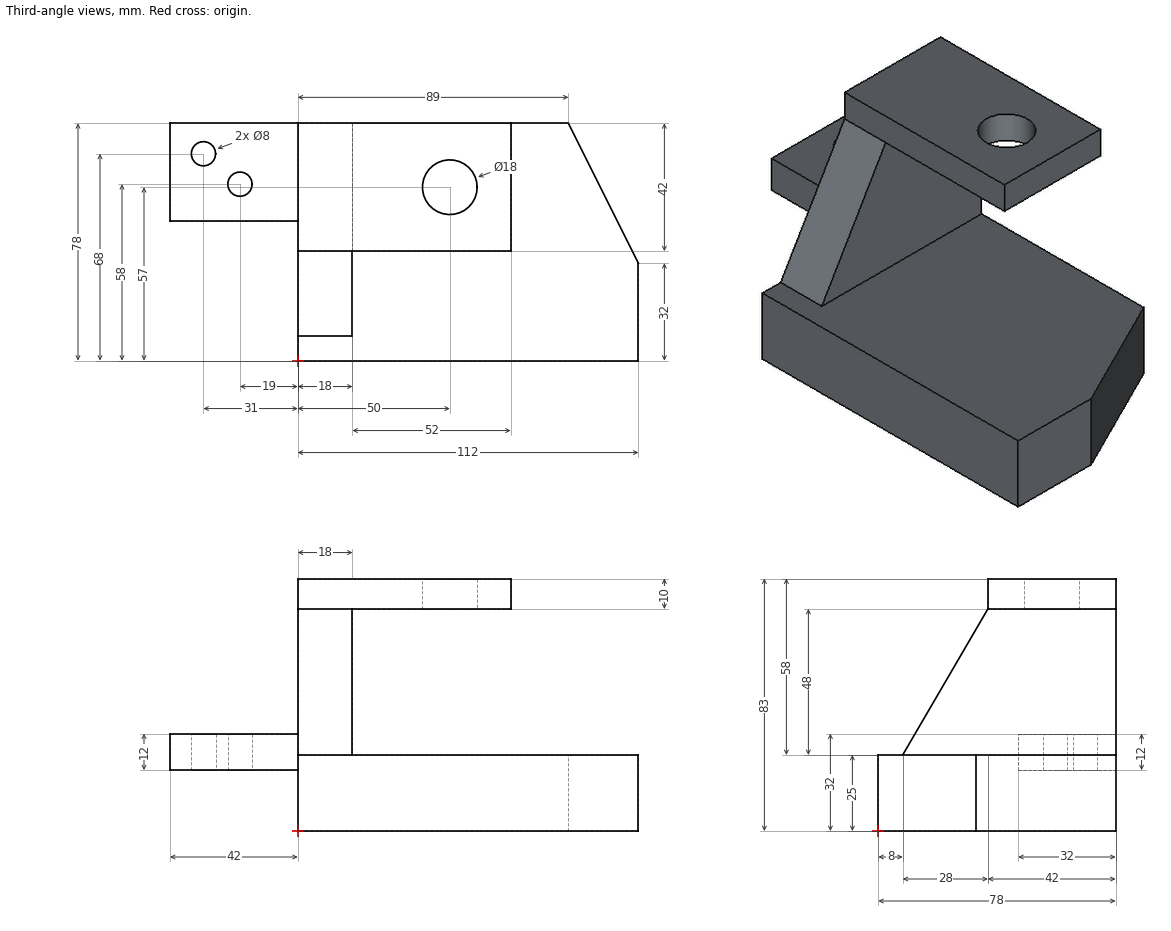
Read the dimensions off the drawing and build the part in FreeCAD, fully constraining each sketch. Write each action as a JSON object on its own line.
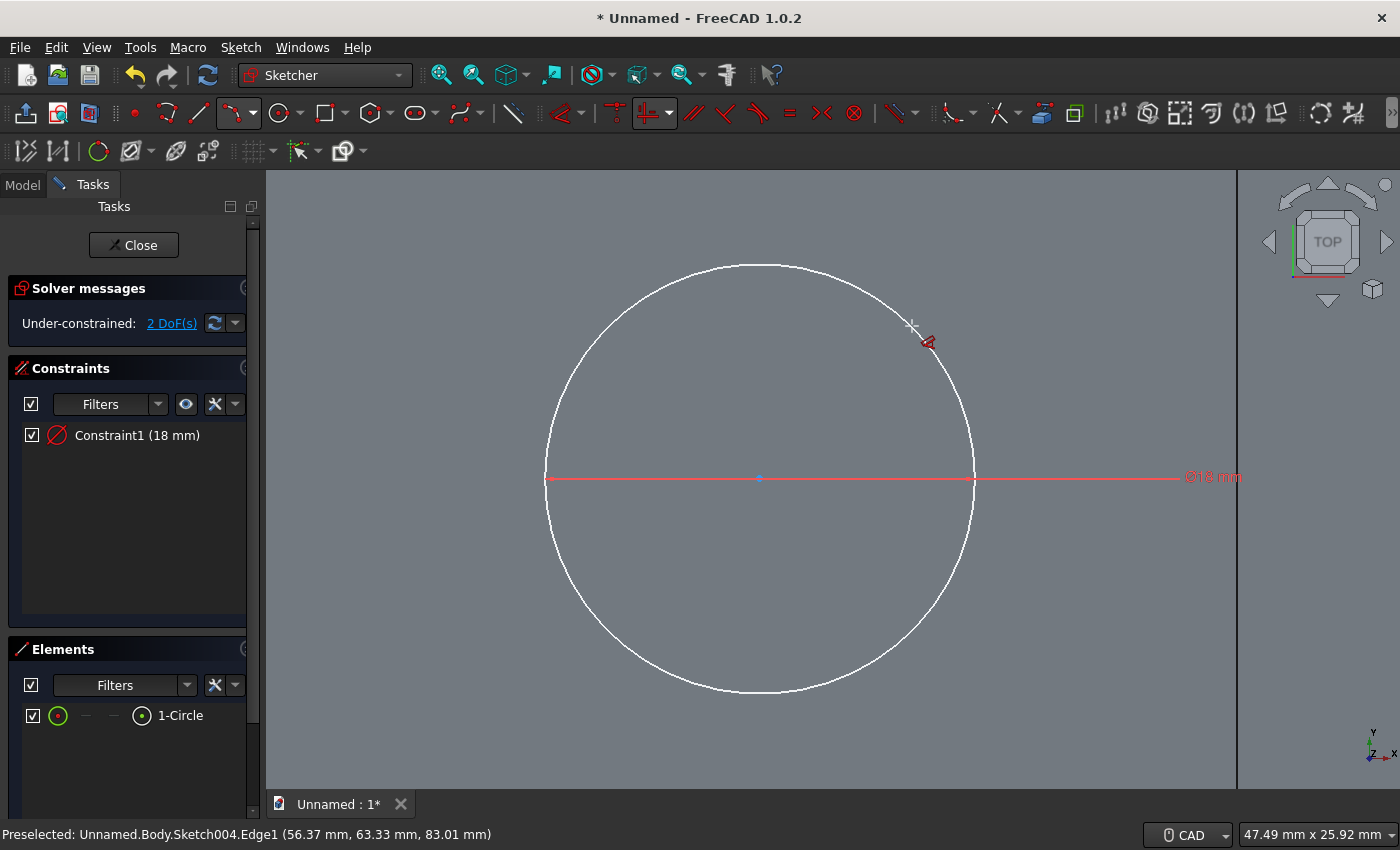
{"action": "left_click", "coordinate": [760, 479]}
{"action": "left_click", "coordinate": [527, 445]}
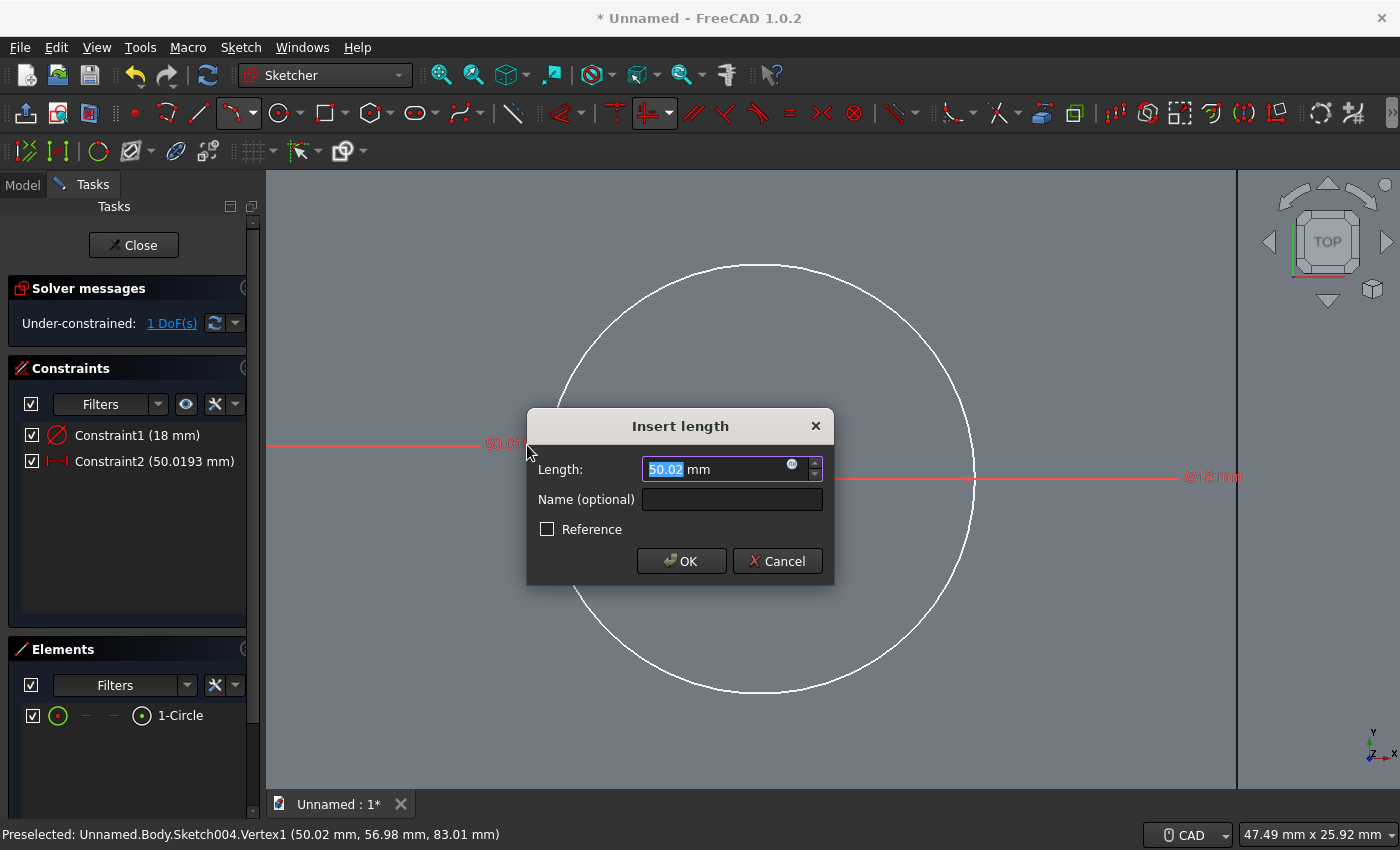
{"action": "type", "text": "50"}
{"action": "key", "text": "Return"}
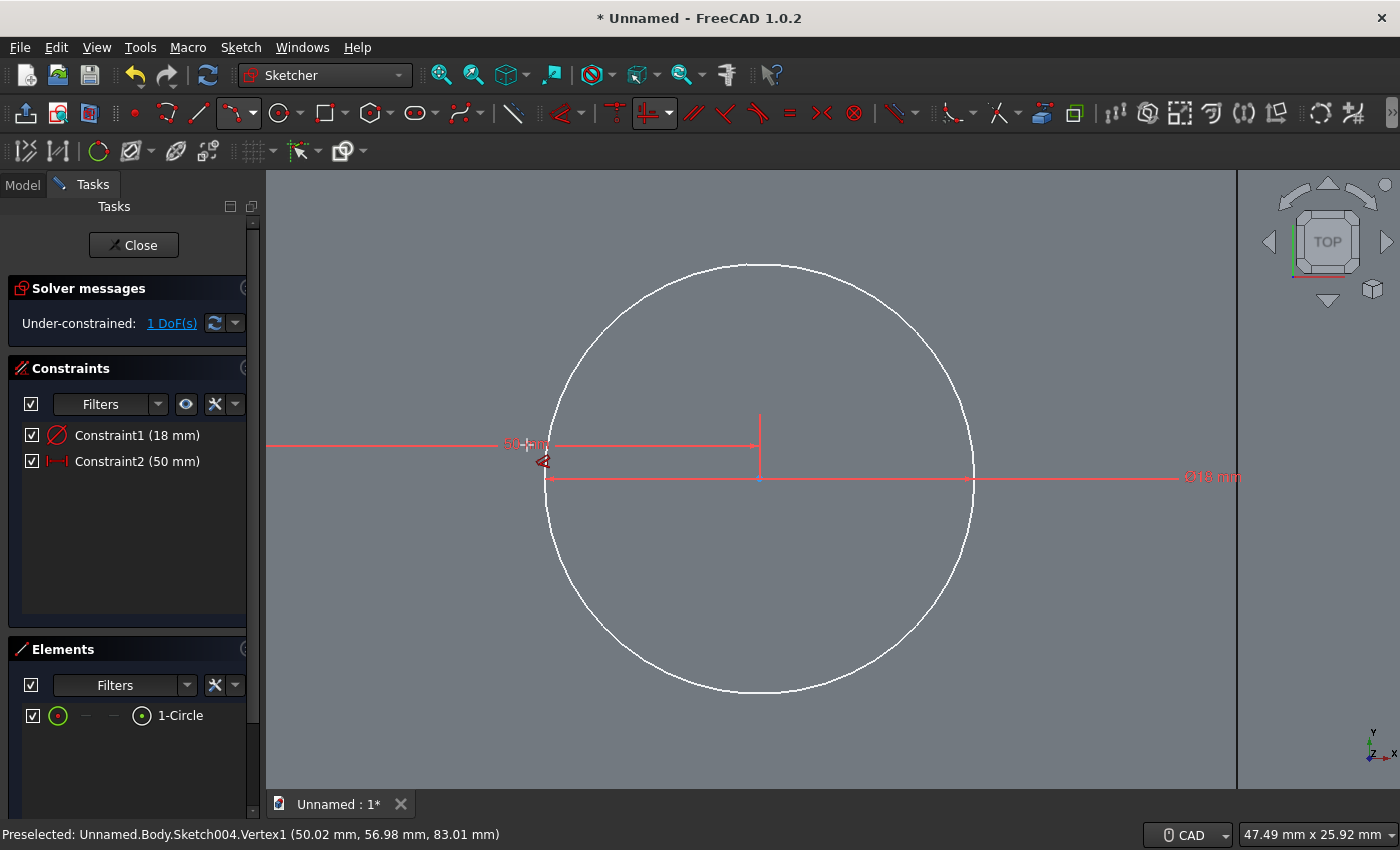
{"action": "left_click", "coordinate": [760, 479]}
{"action": "left_click", "coordinate": [794, 620]}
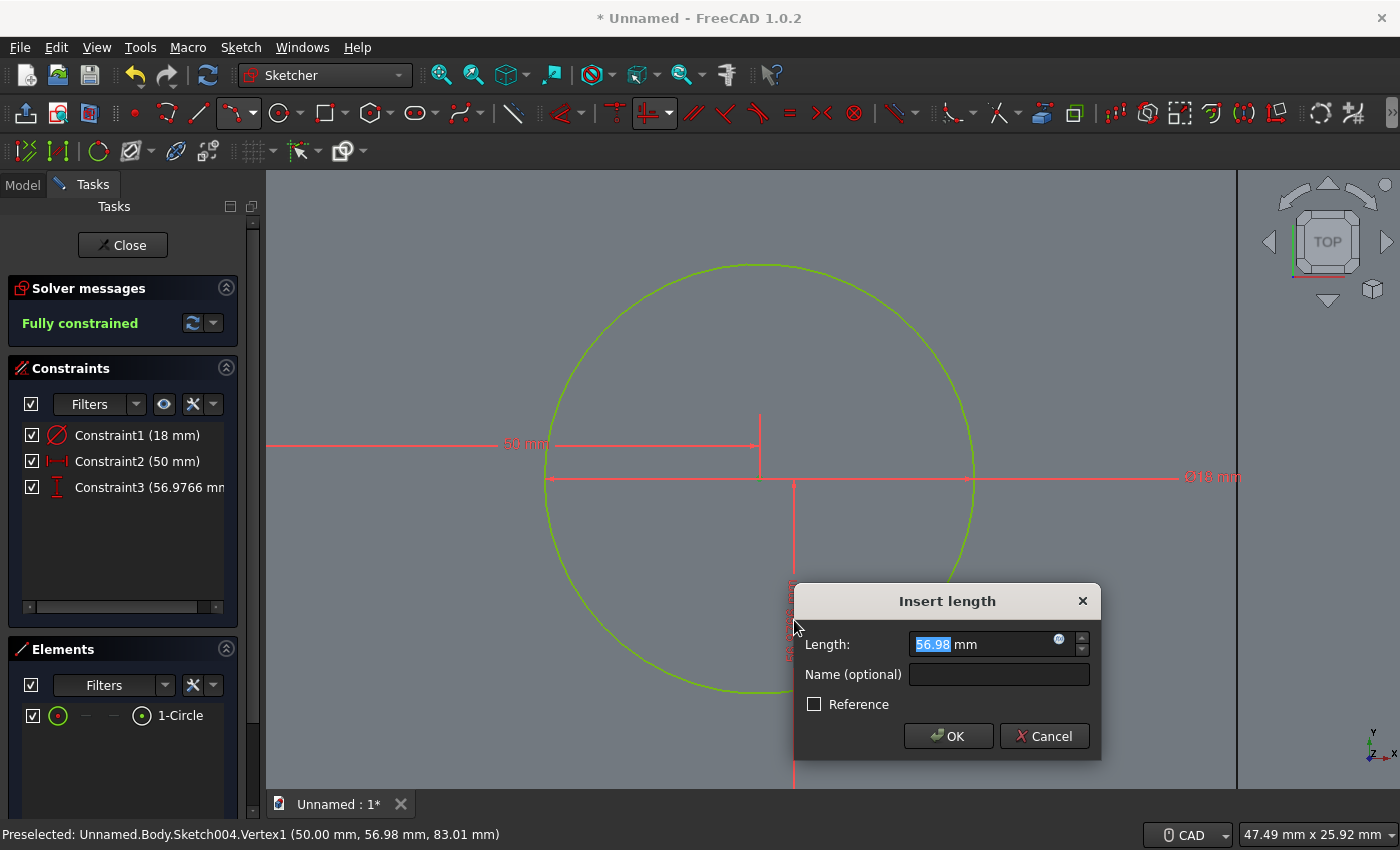
{"action": "type", "text": "57"}
{"action": "key", "text": "Return"}
{"action": "key", "text": "Escape"}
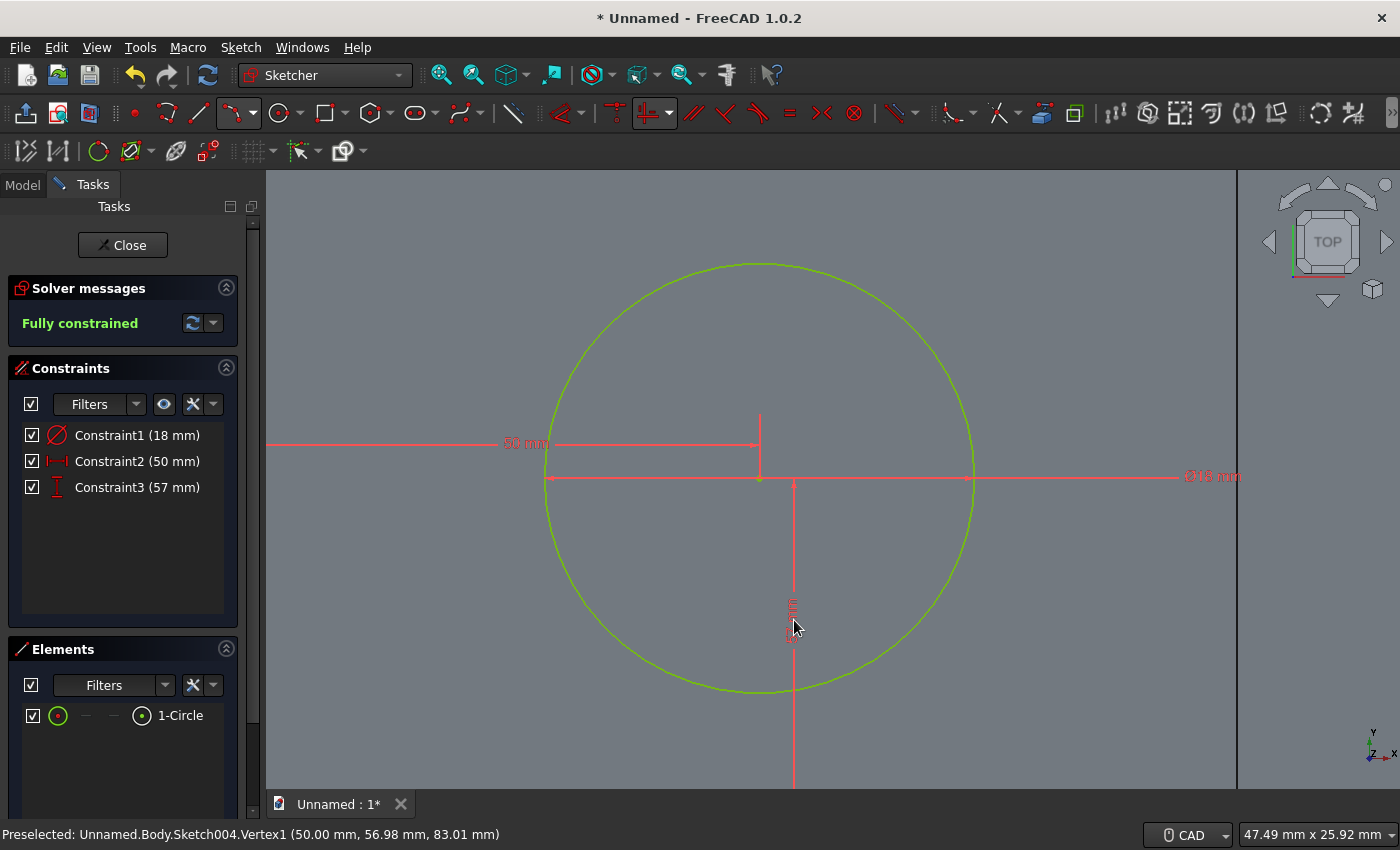
{"action": "left_click", "coordinate": [123, 245]}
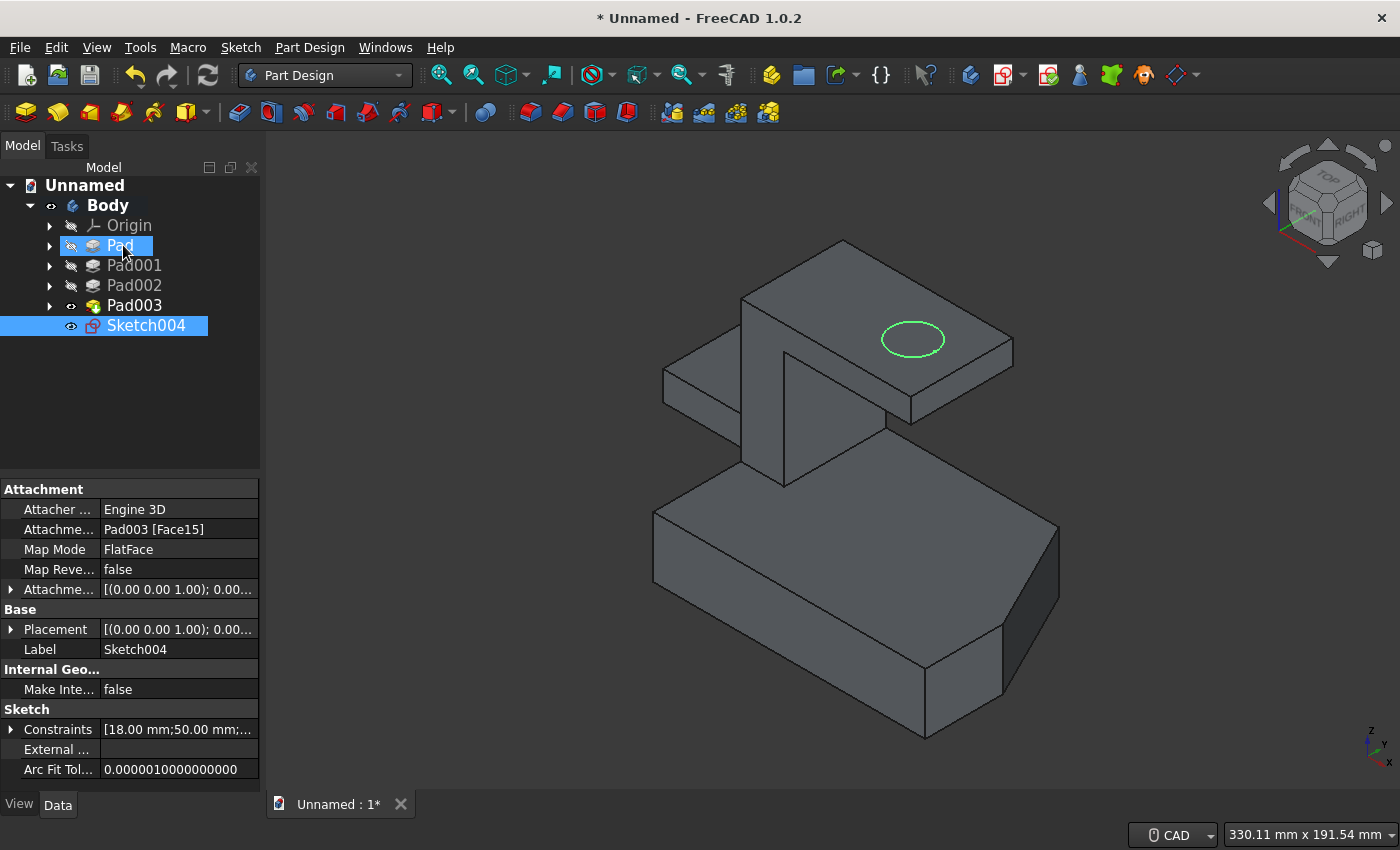
{"action": "left_click", "coordinate": [240, 112]}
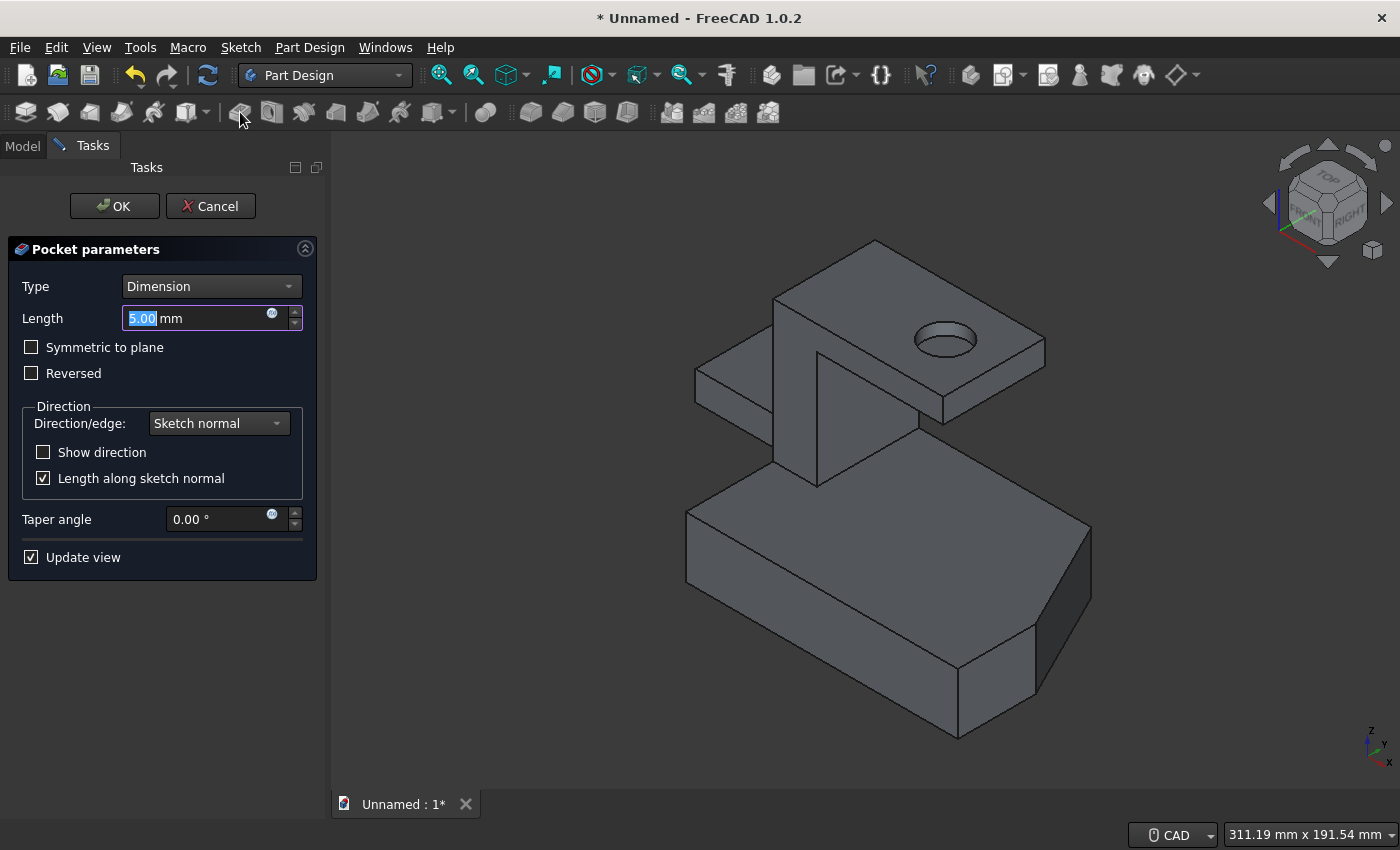
{"action": "type", "text": "10"}
{"action": "key", "text": "Tab"}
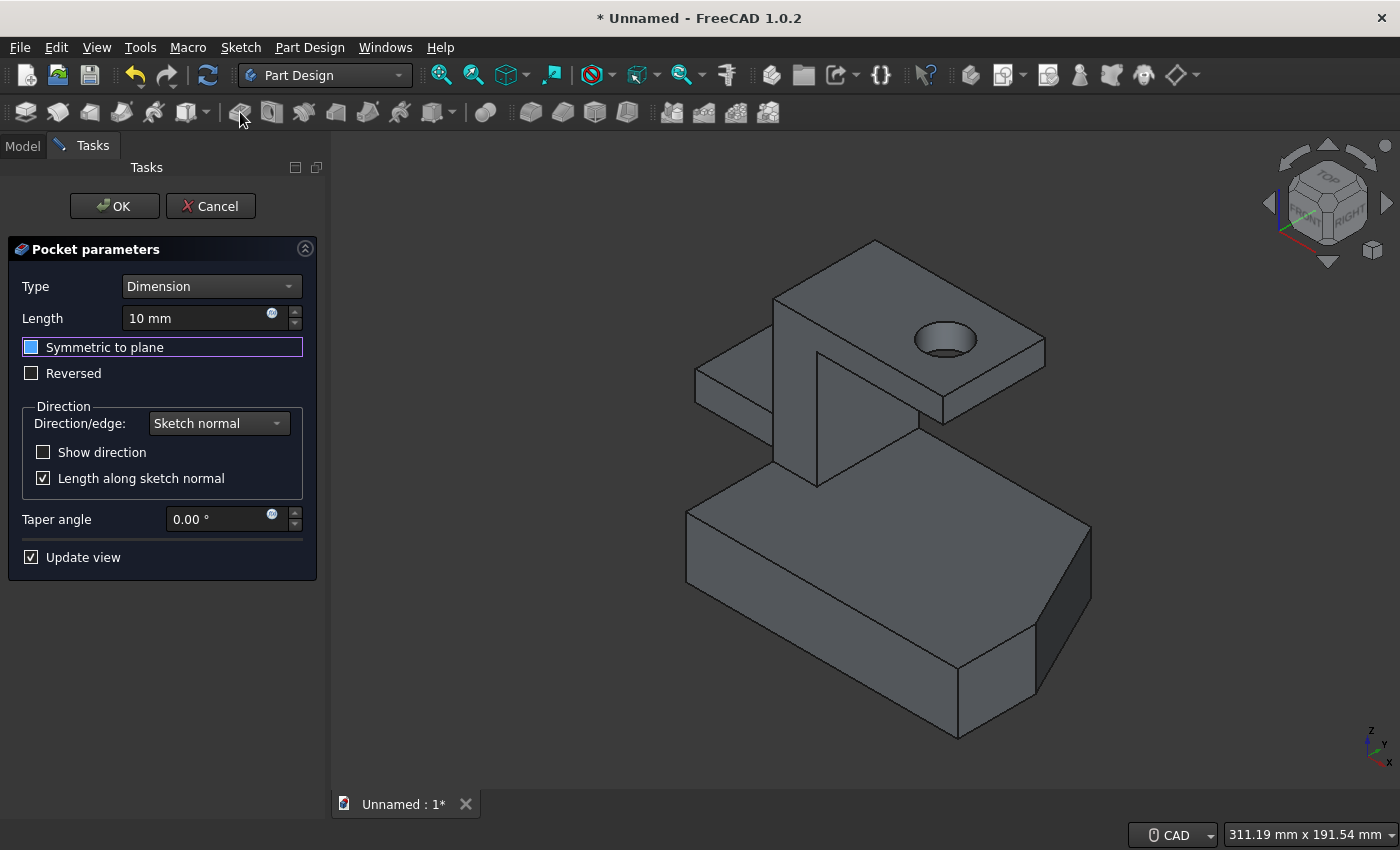
{"action": "left_click", "coordinate": [115, 206]}